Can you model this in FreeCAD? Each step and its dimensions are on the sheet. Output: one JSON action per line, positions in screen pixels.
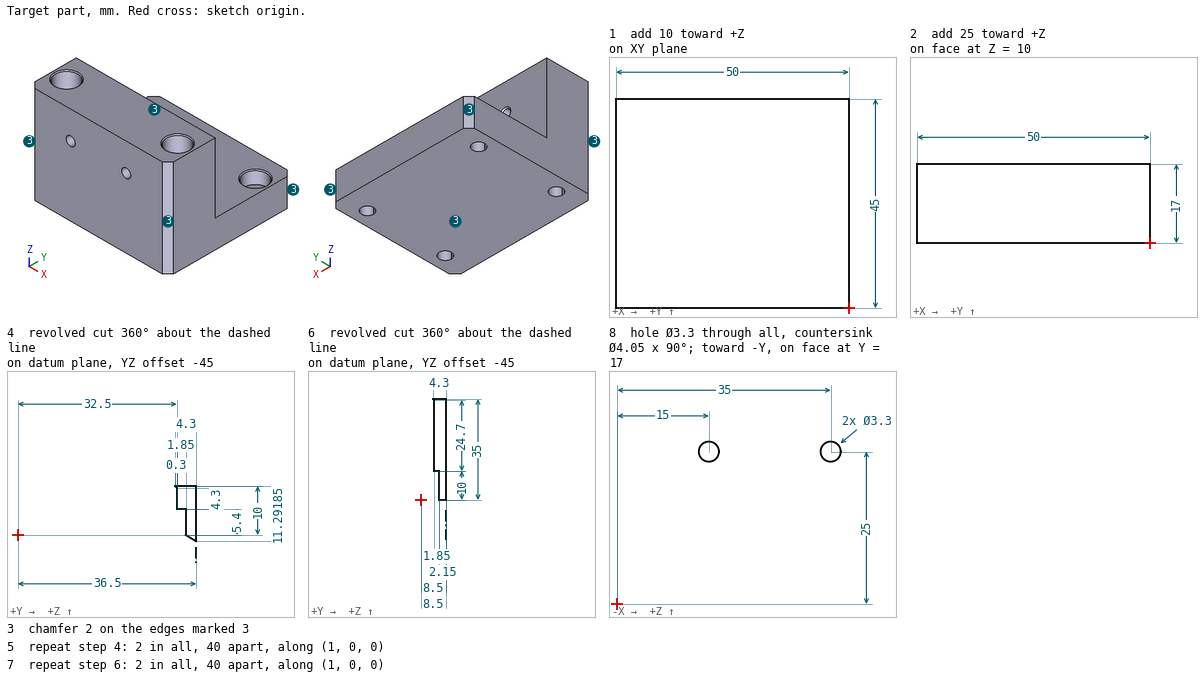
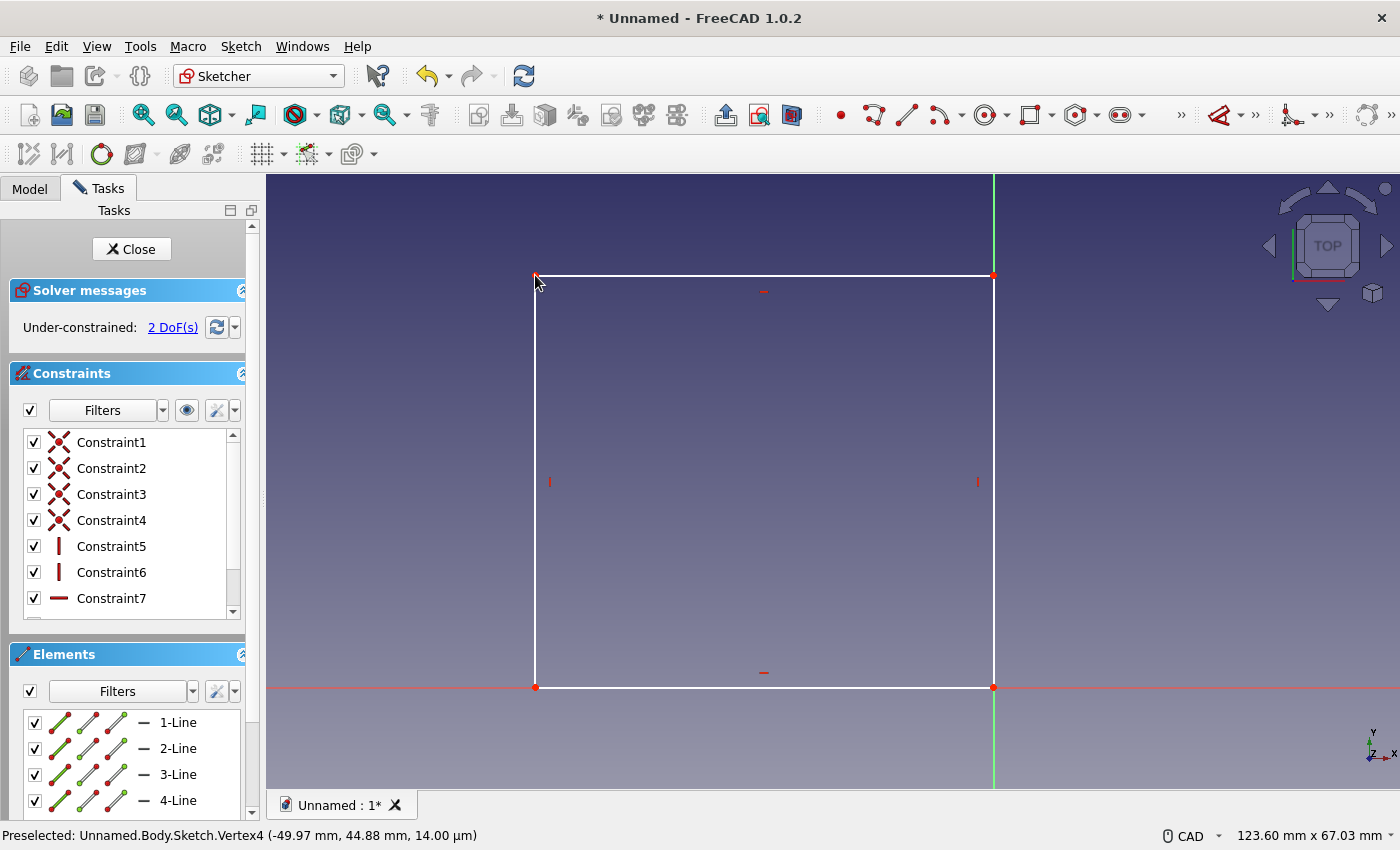
{"action": "left_click", "coordinate": [994, 564]}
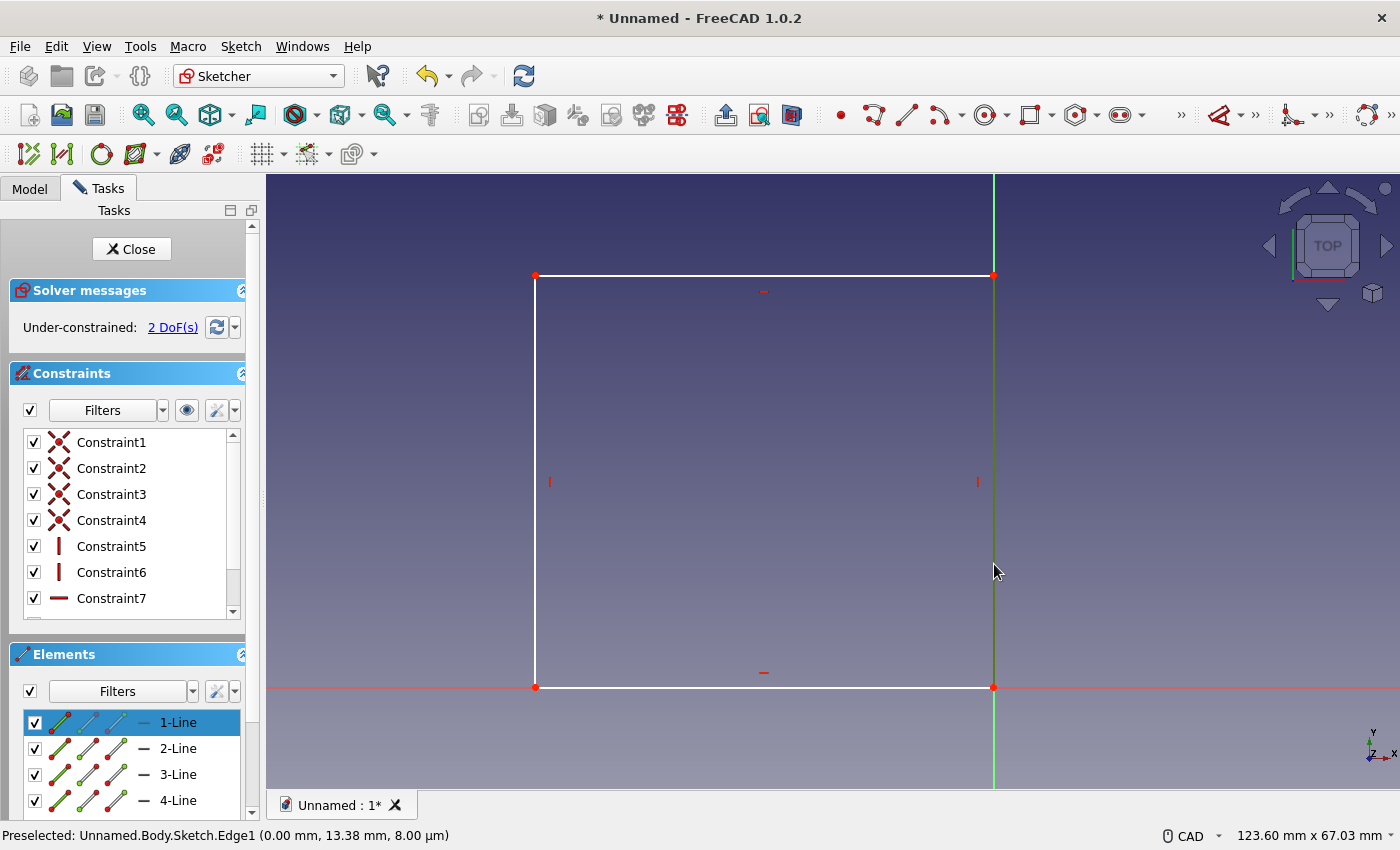
{"action": "key", "text": "i"}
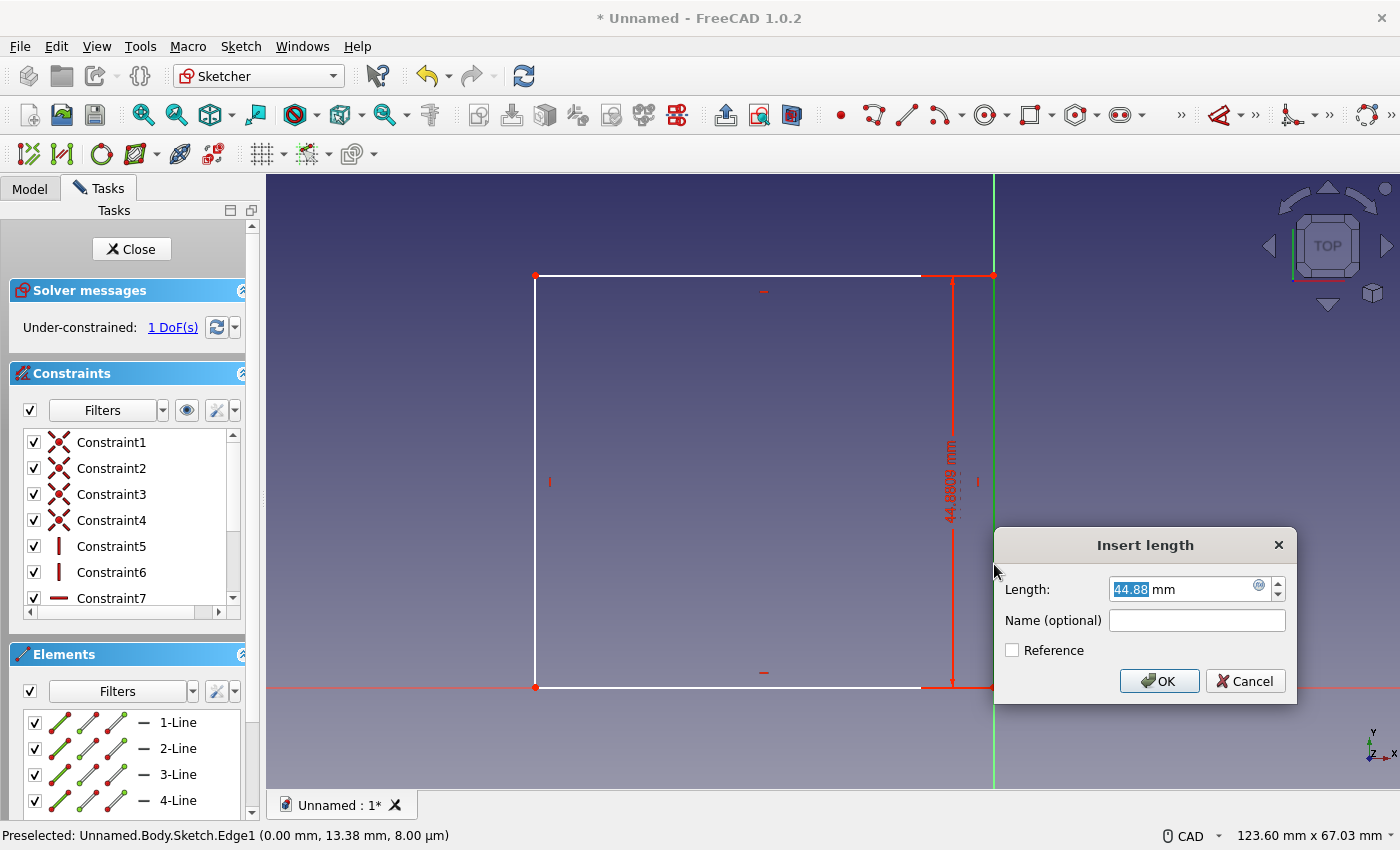
{"action": "type", "text": "45"}
{"action": "key", "text": "Return"}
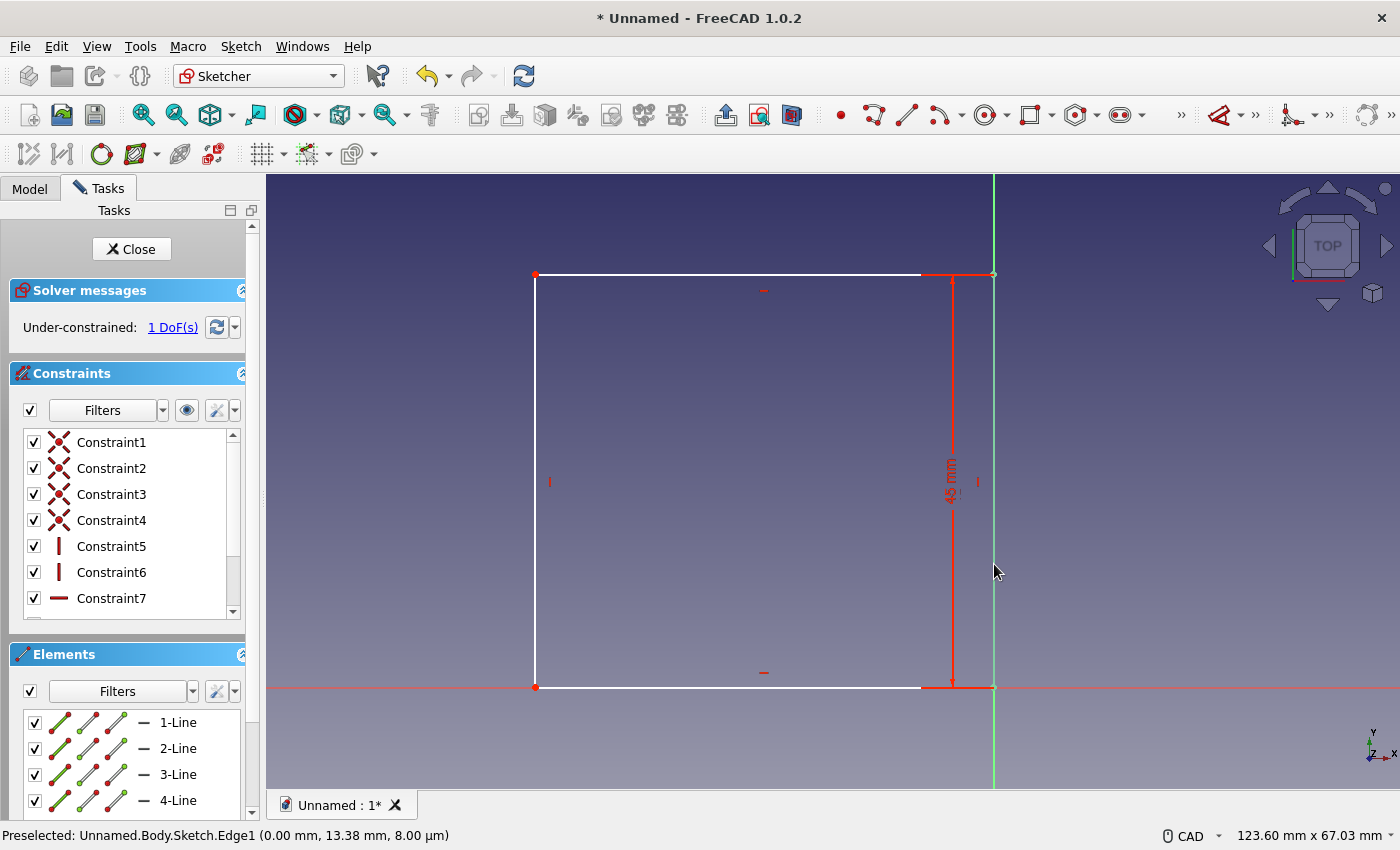
{"action": "left_click", "coordinate": [856, 275]}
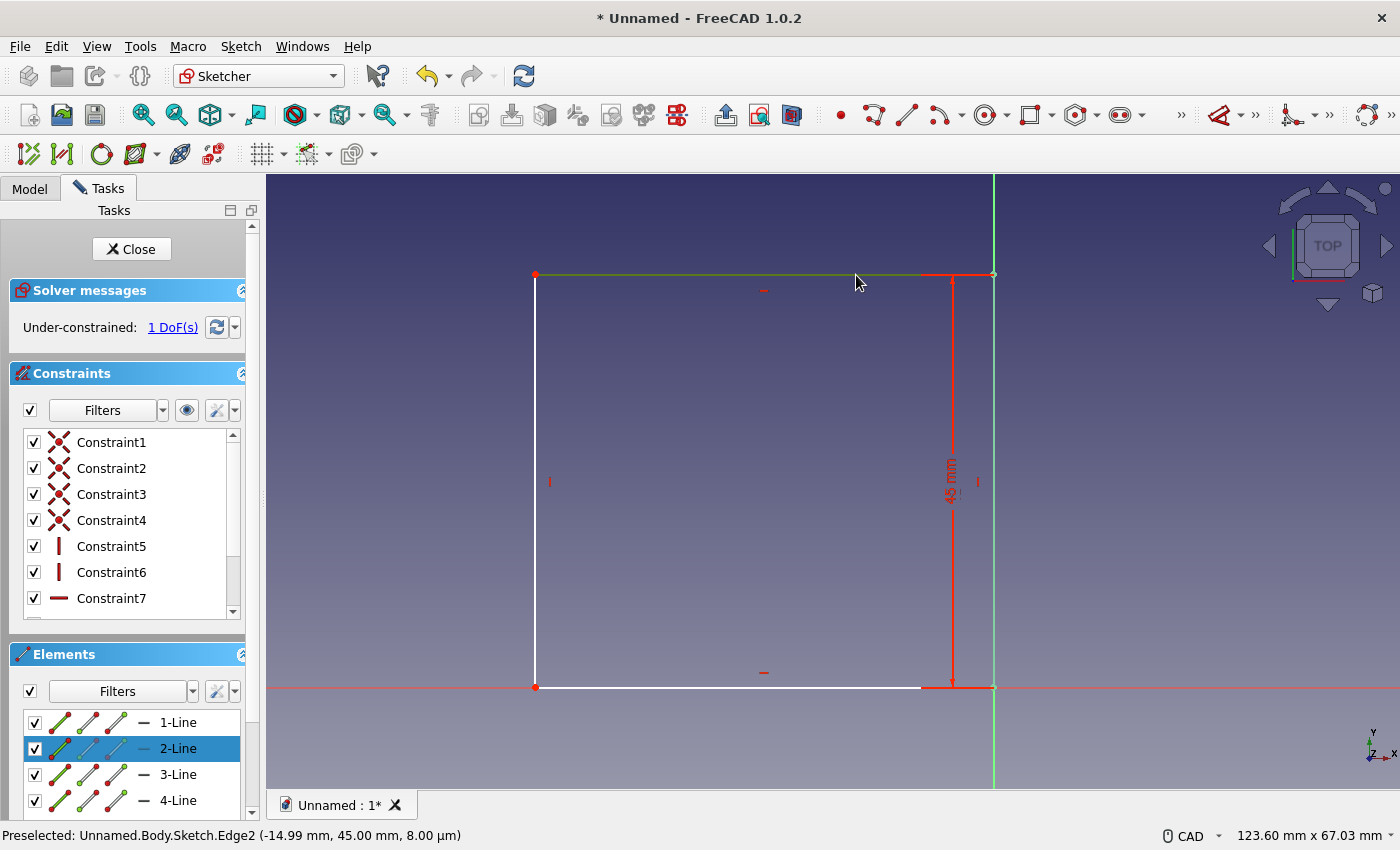
{"action": "key", "text": "l"}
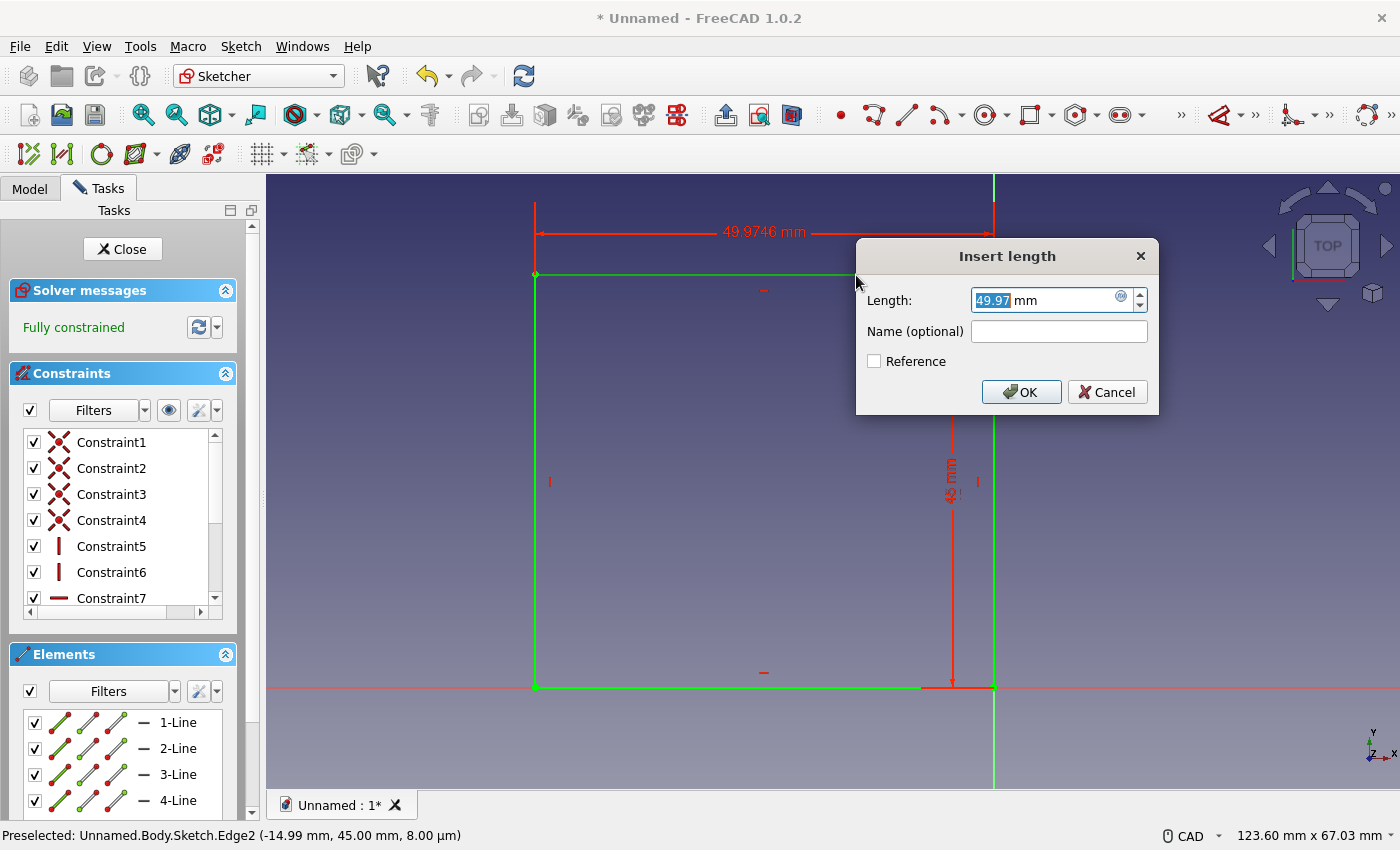
{"action": "type", "text": "50"}
{"action": "key", "text": "Return"}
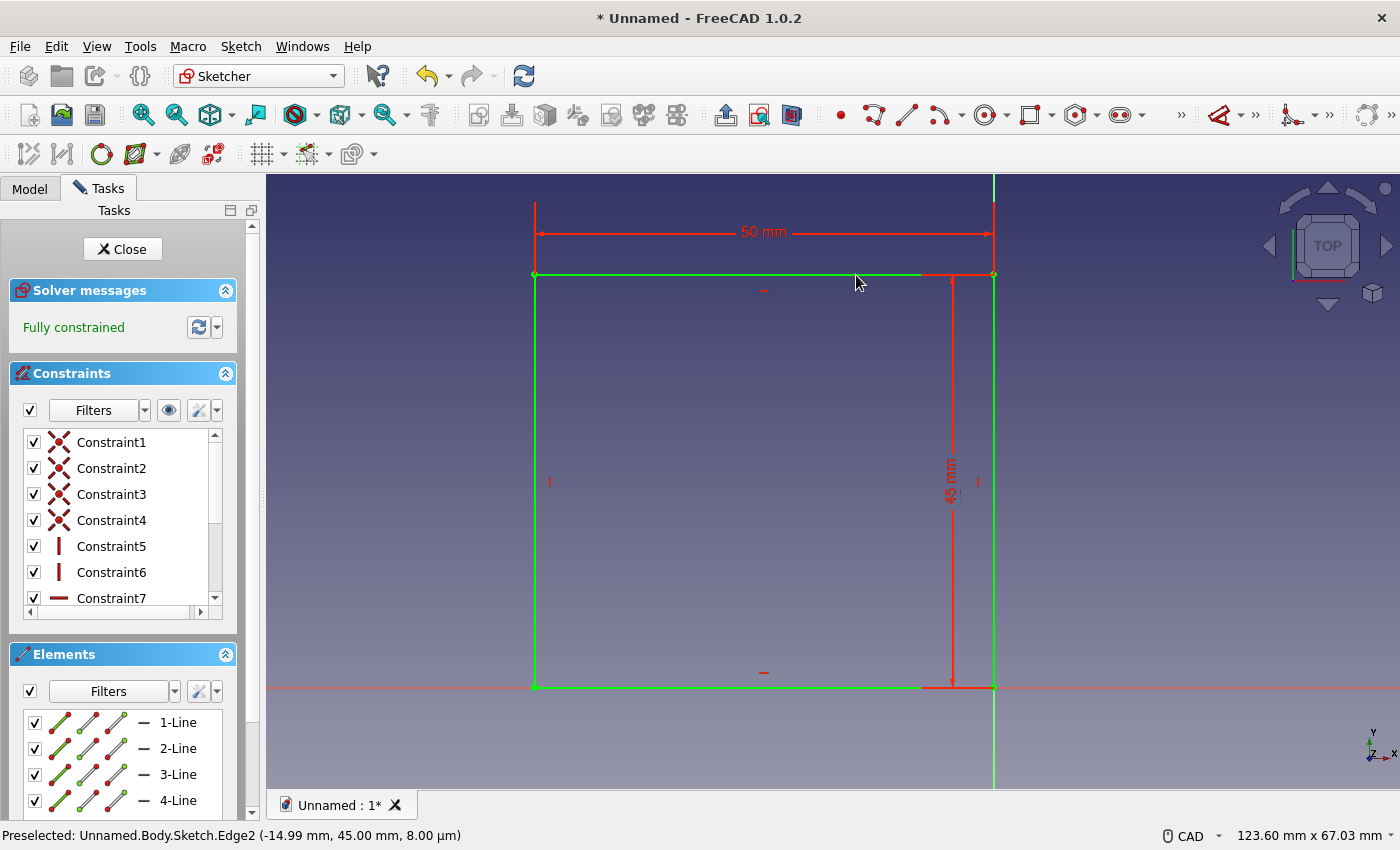
{"action": "left_click", "coordinate": [123, 249]}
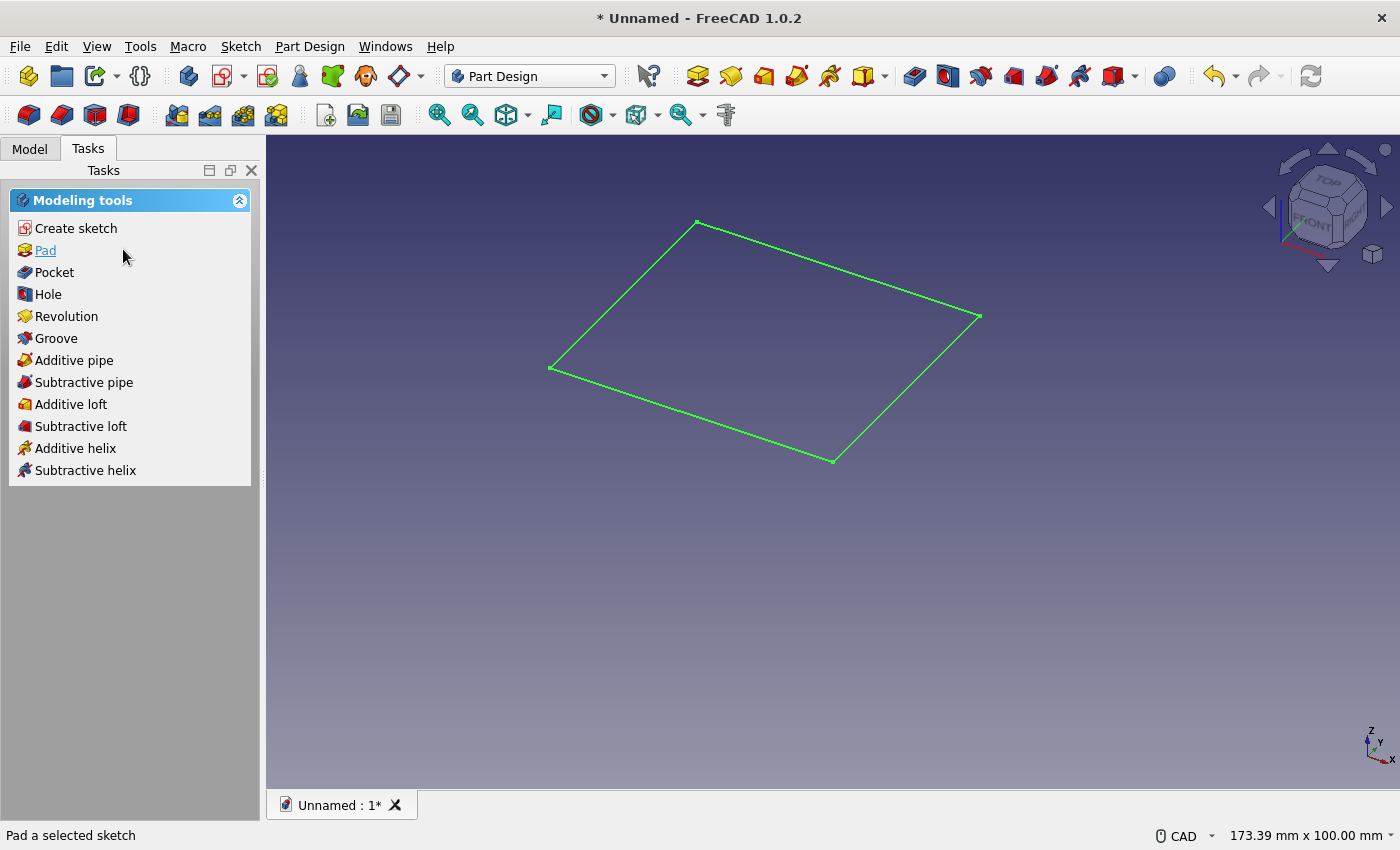
{"action": "left_click", "coordinate": [698, 76]}